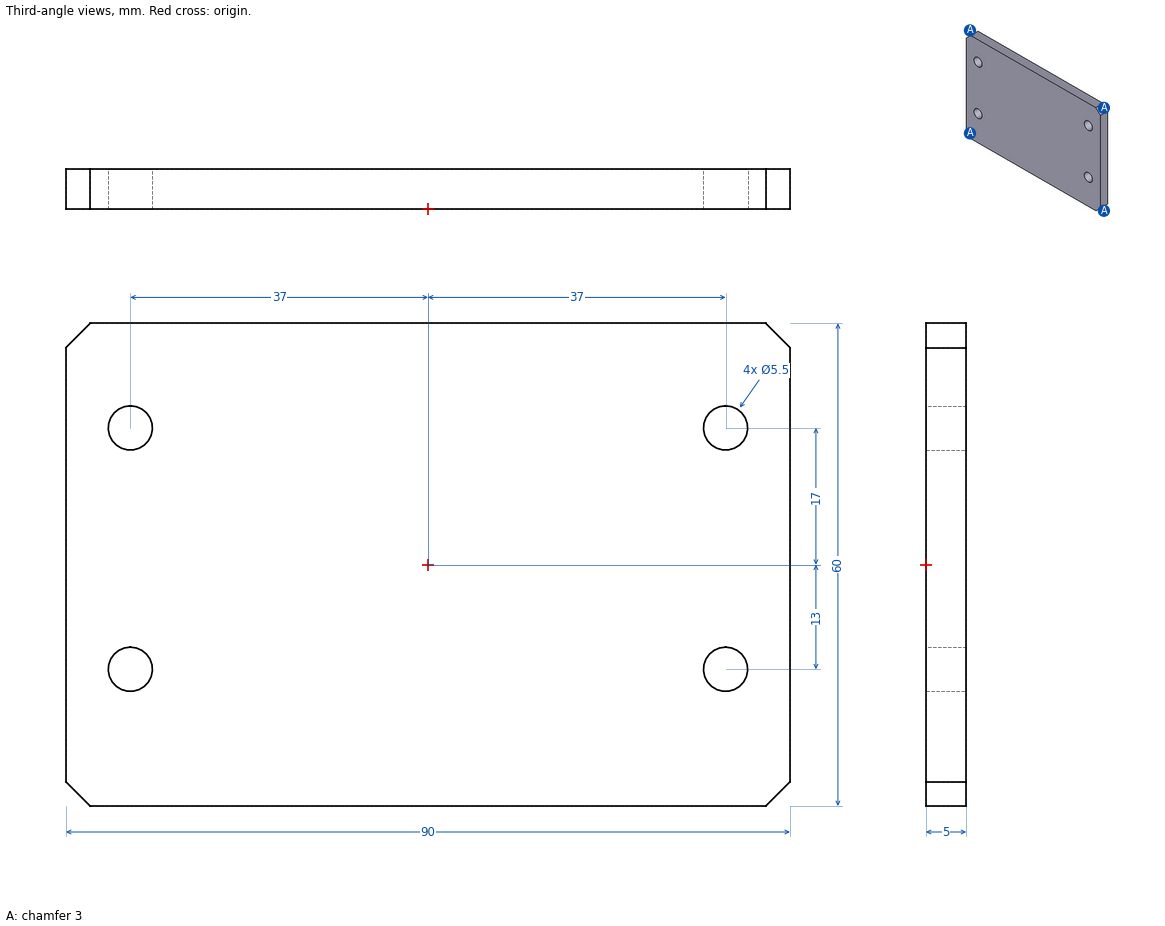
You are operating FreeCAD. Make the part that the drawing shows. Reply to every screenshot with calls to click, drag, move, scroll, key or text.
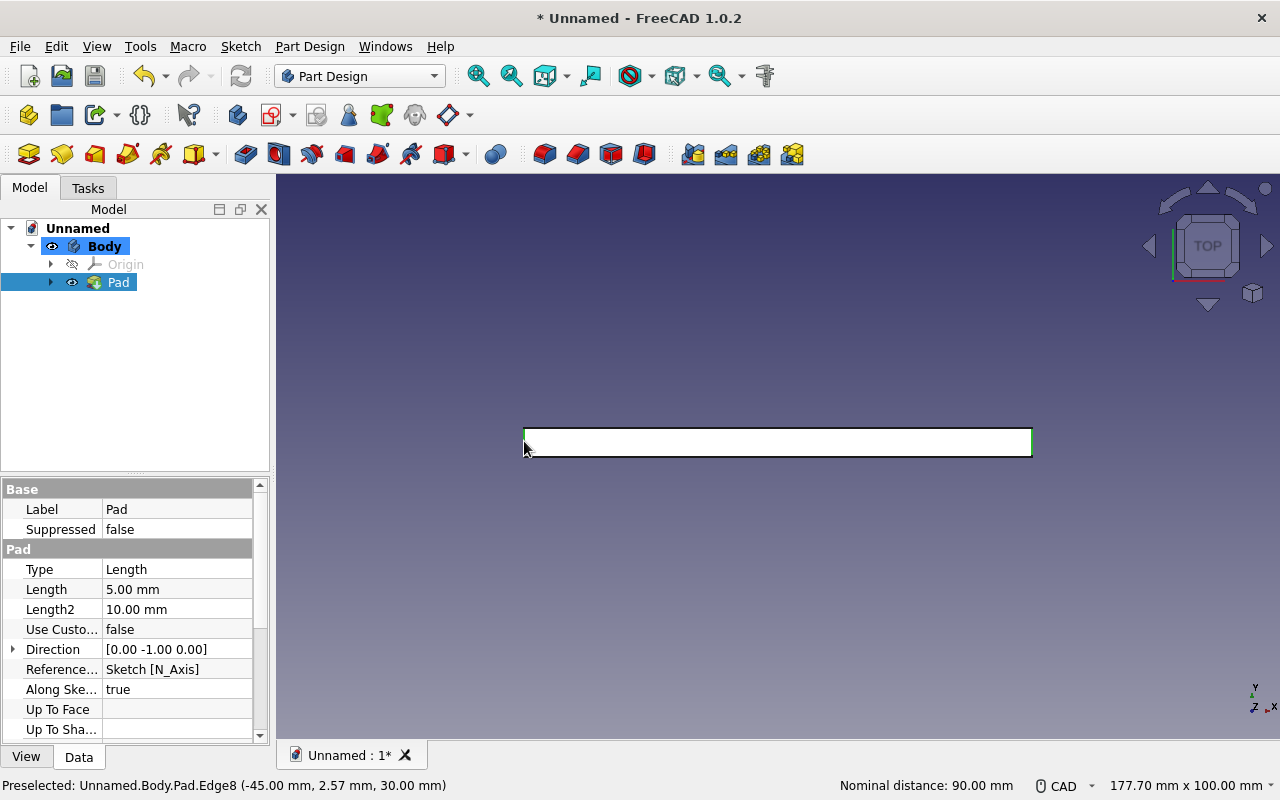
key(1)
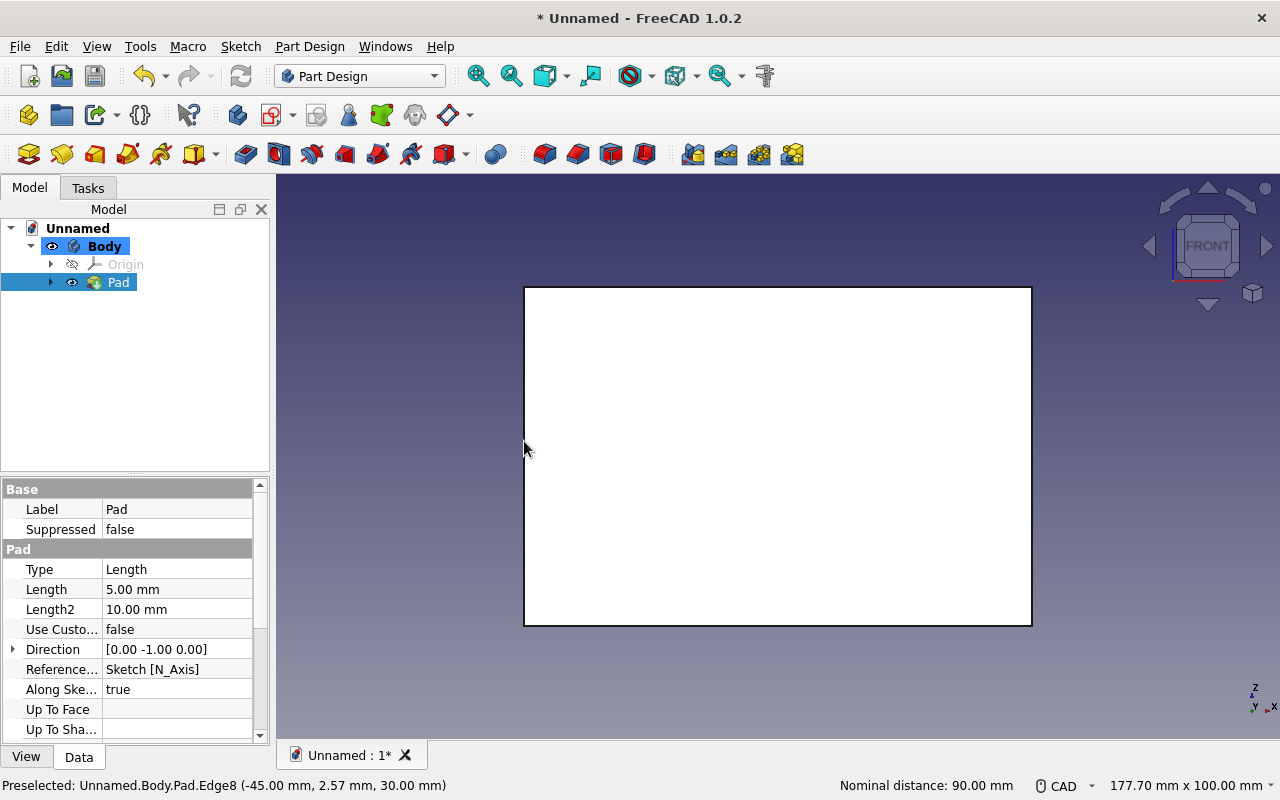
key(3)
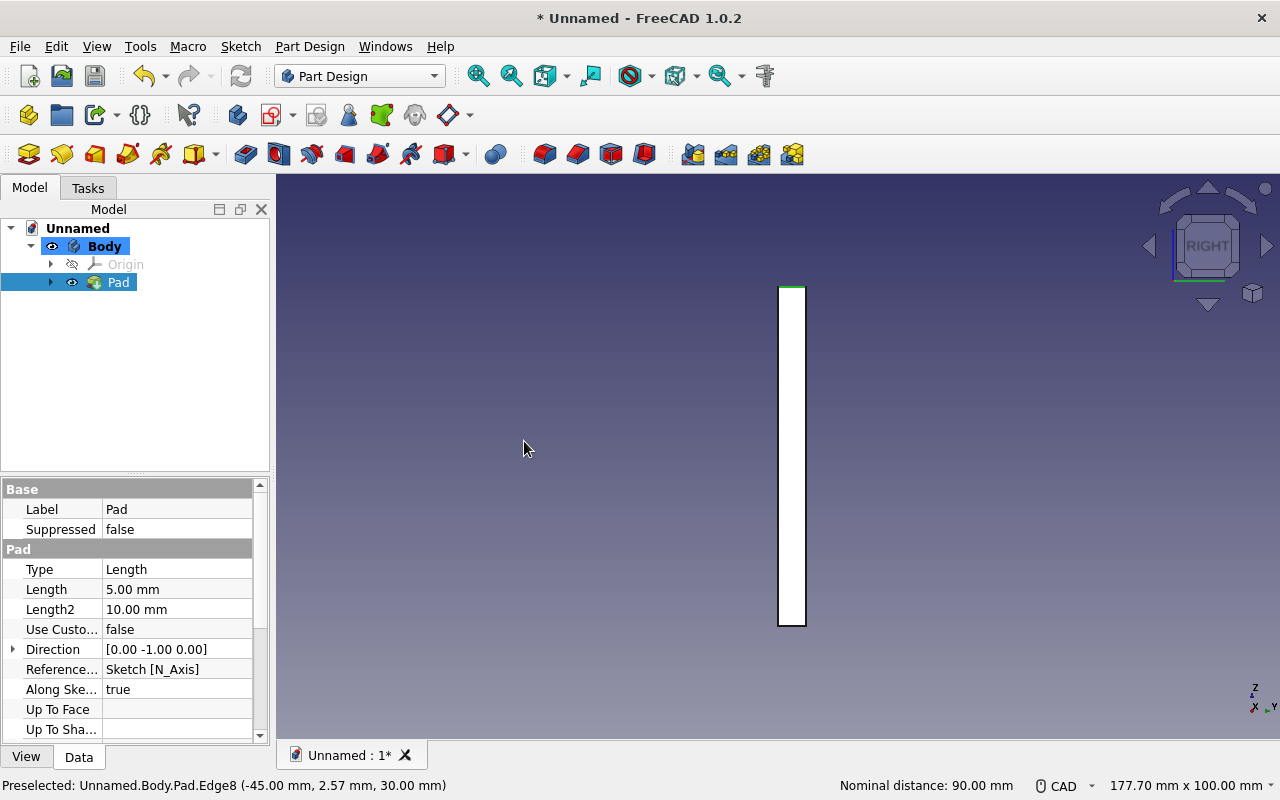
click(792, 625, ctrl)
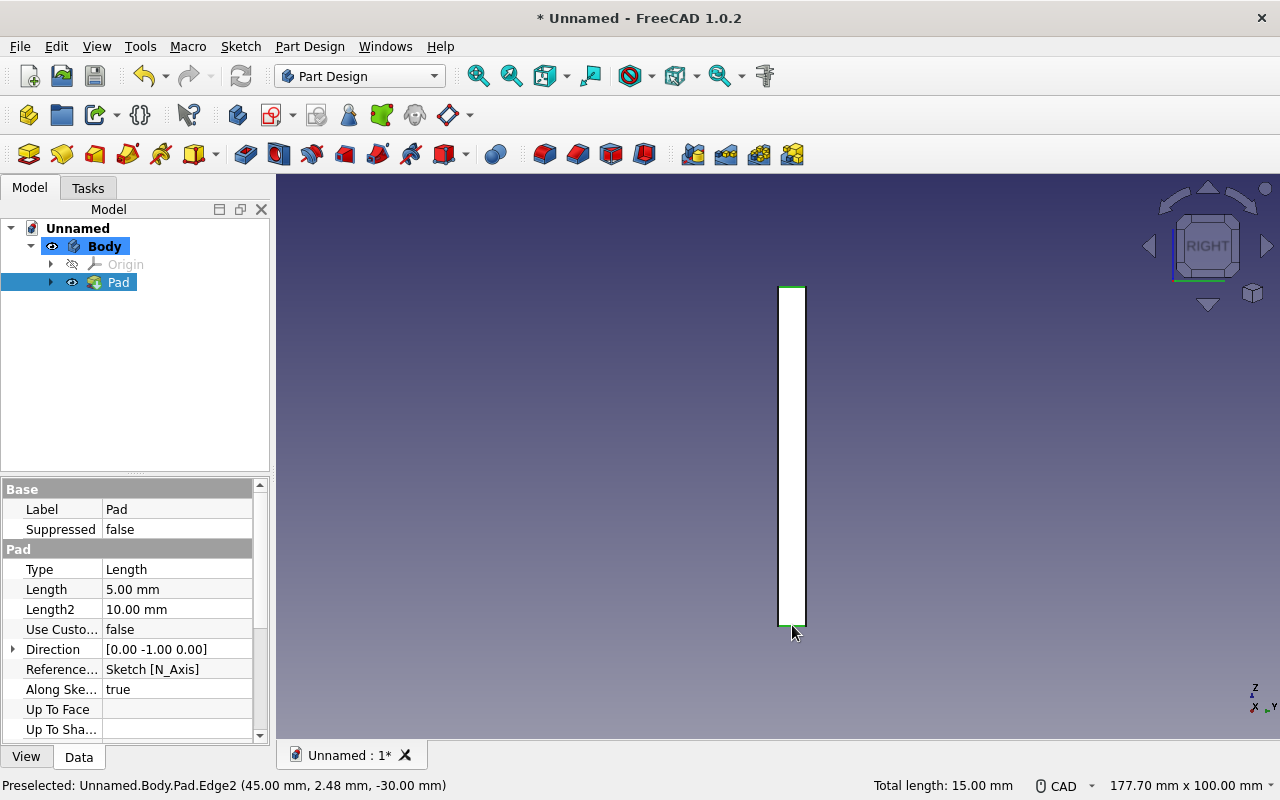
key(5)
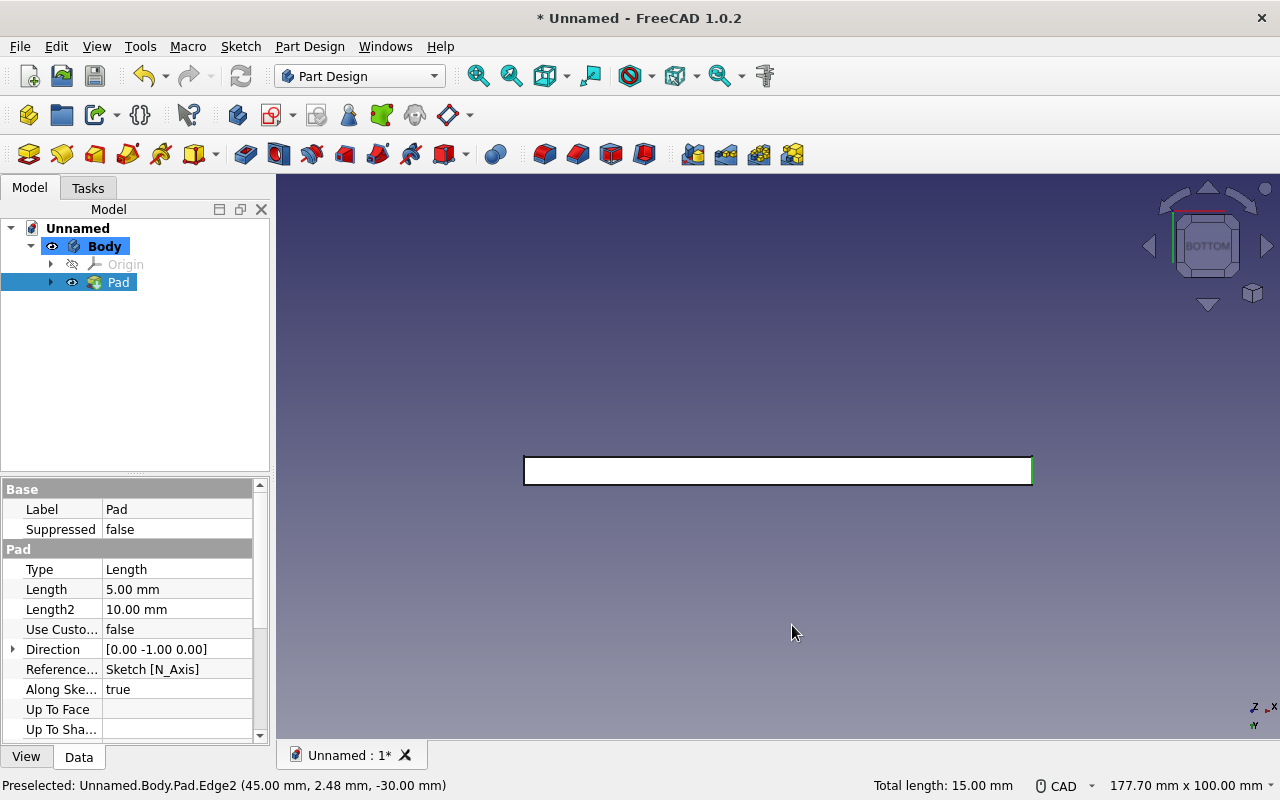
click(524, 470, ctrl)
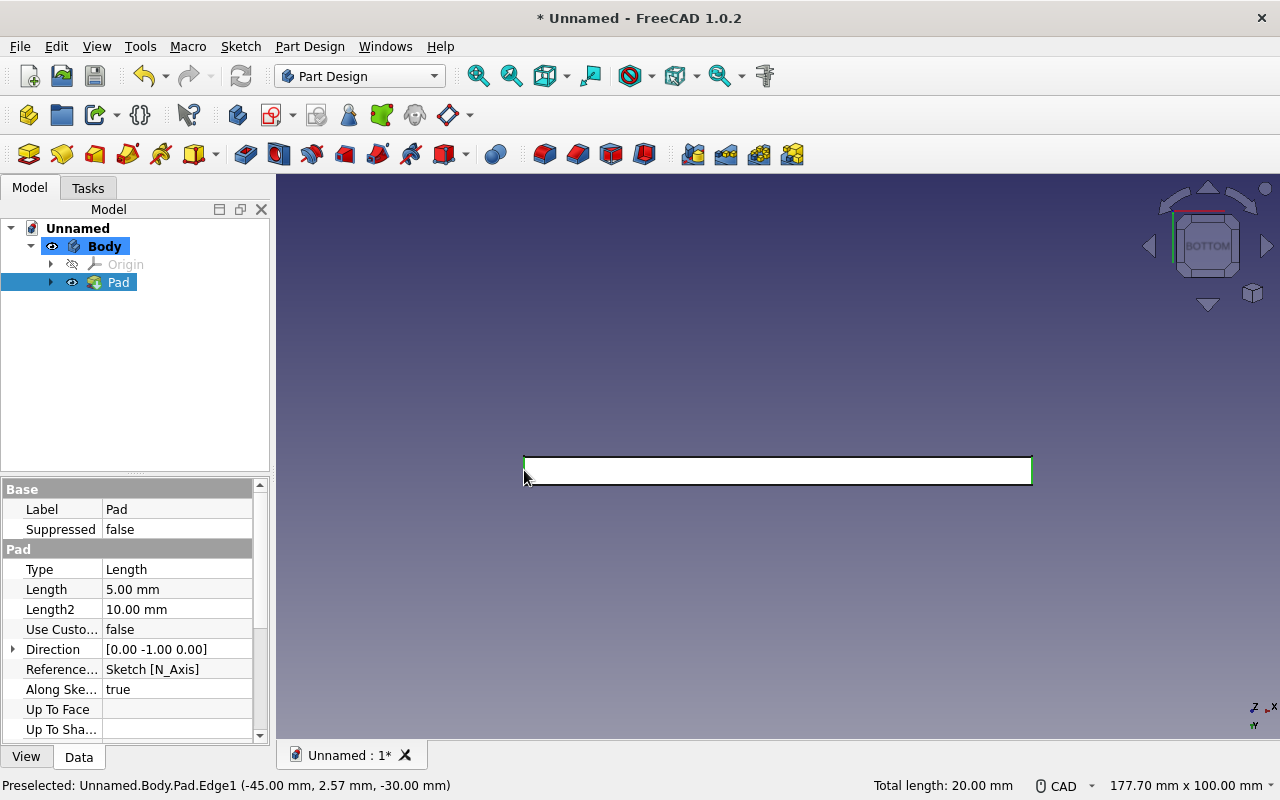
click(578, 154)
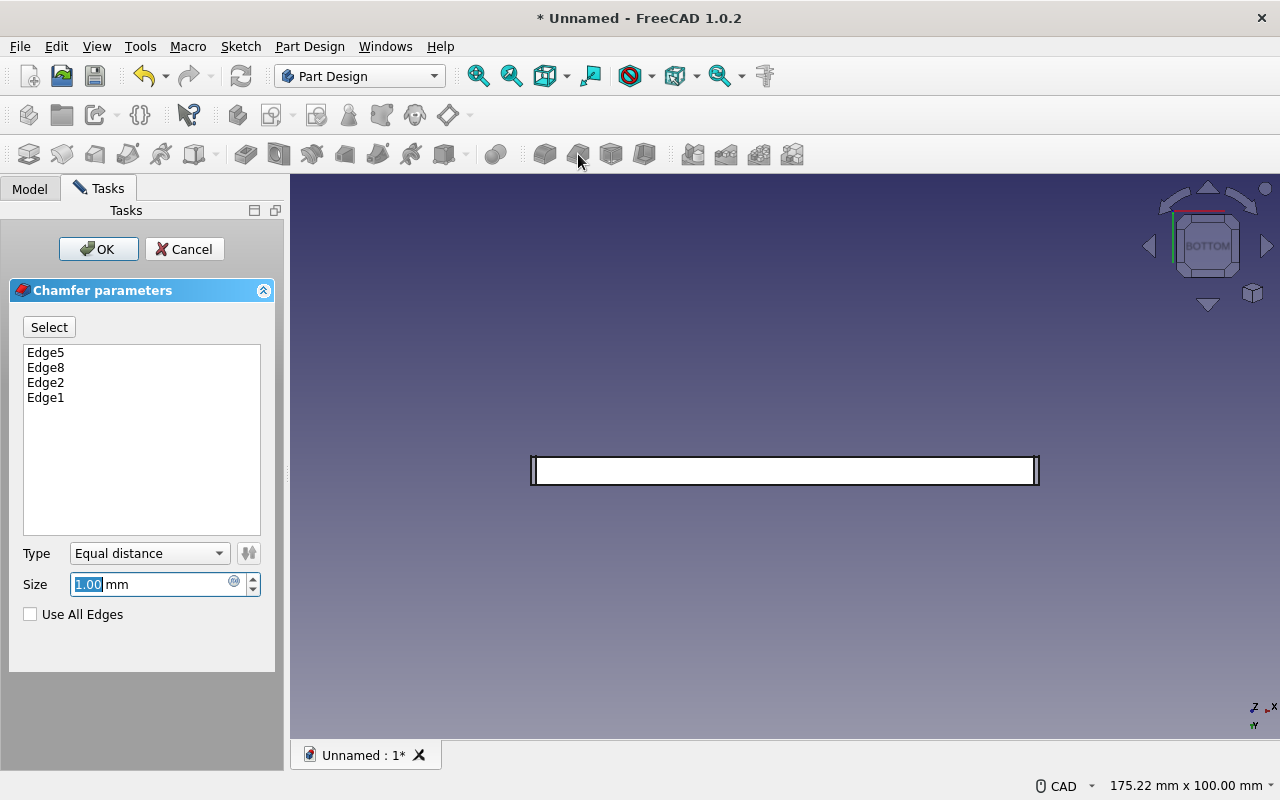
text(3)
key(Tab)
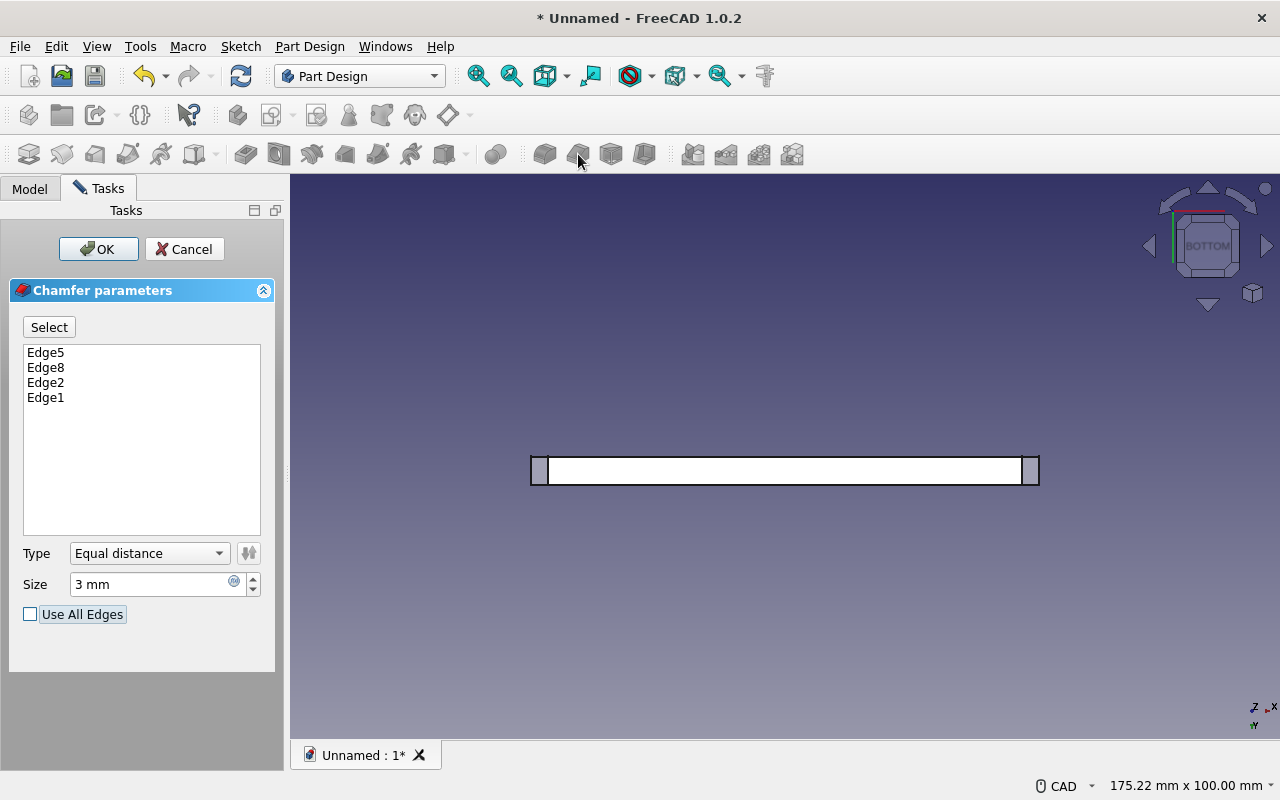
click(99, 249)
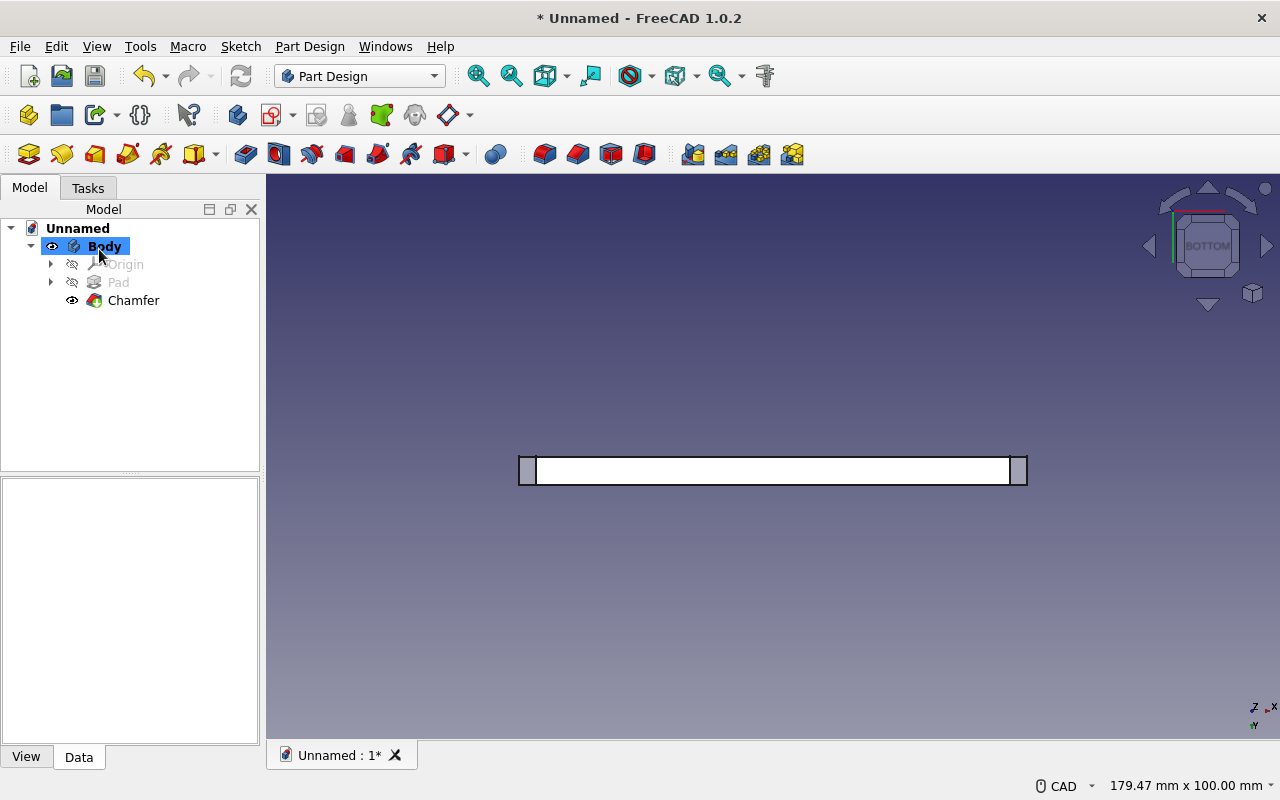
key(4)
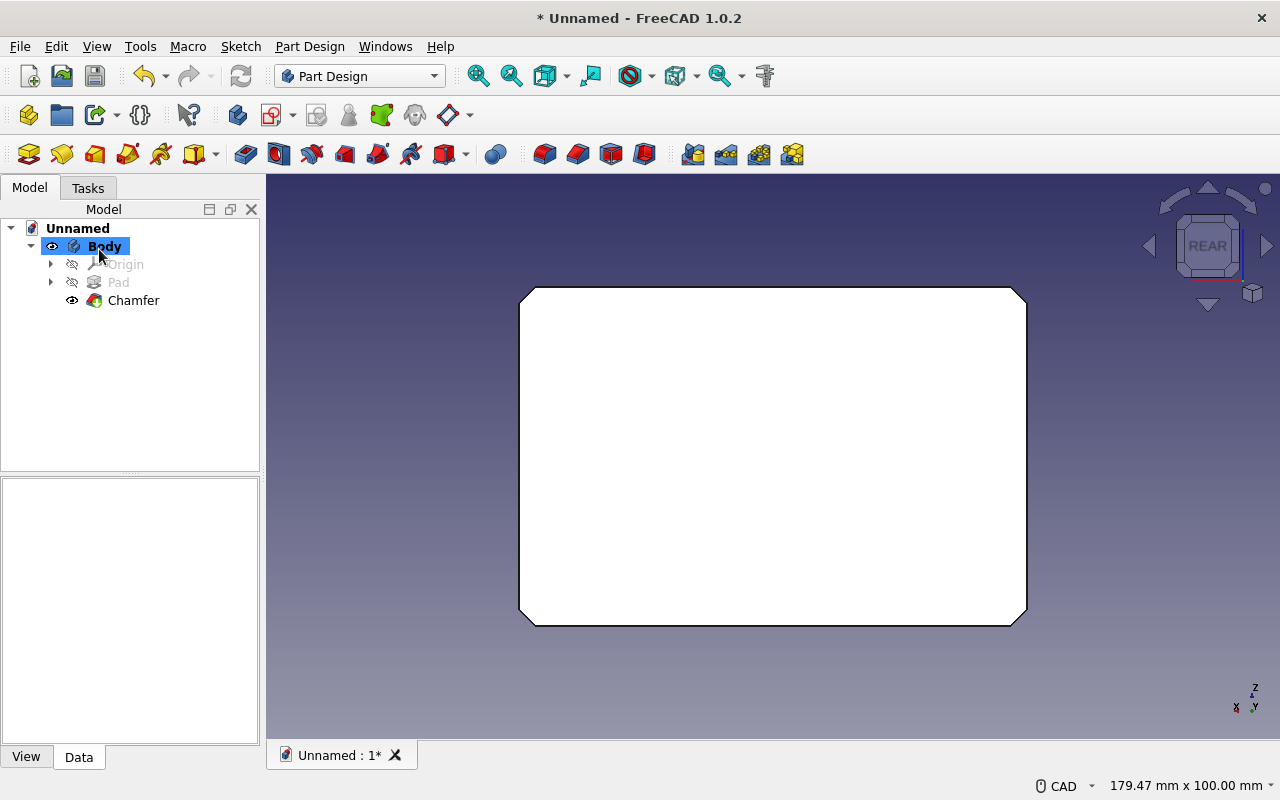
click(700, 455)